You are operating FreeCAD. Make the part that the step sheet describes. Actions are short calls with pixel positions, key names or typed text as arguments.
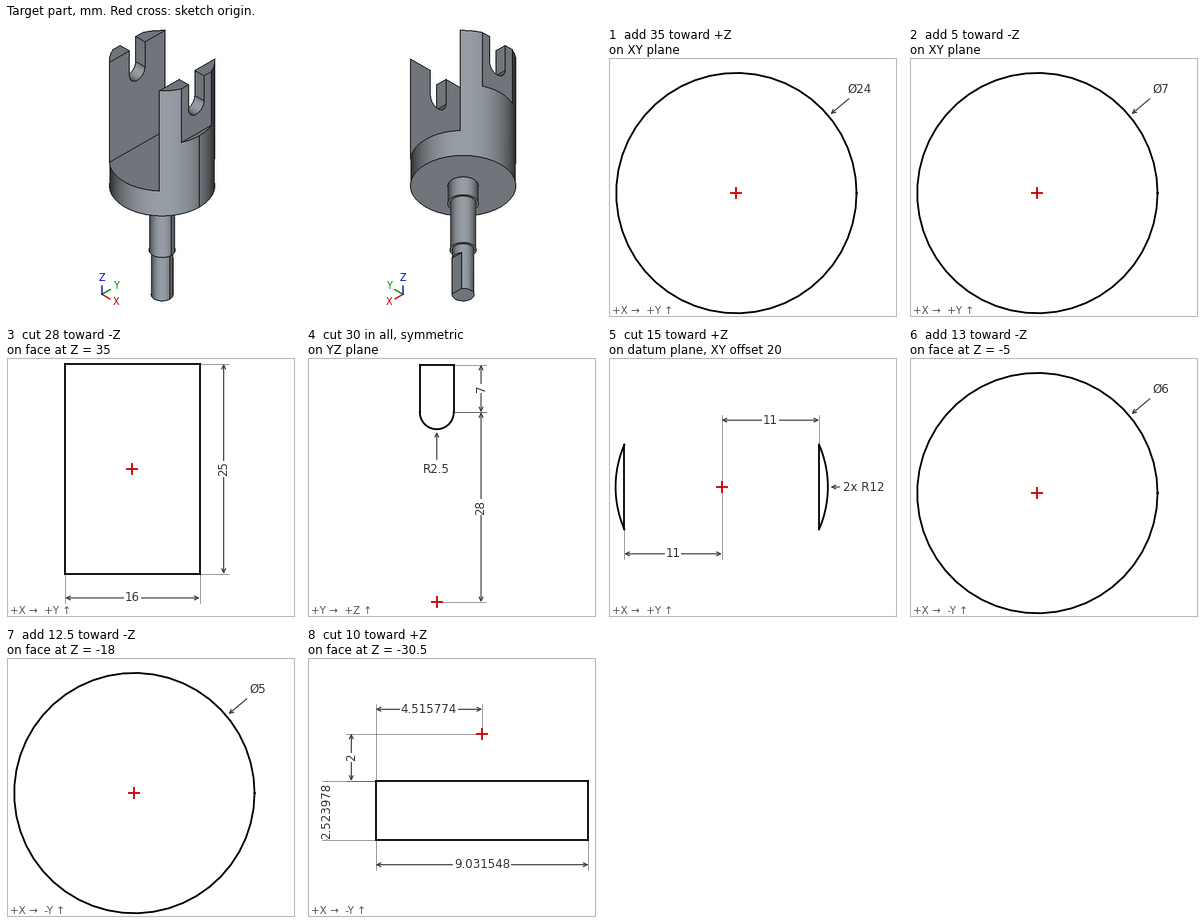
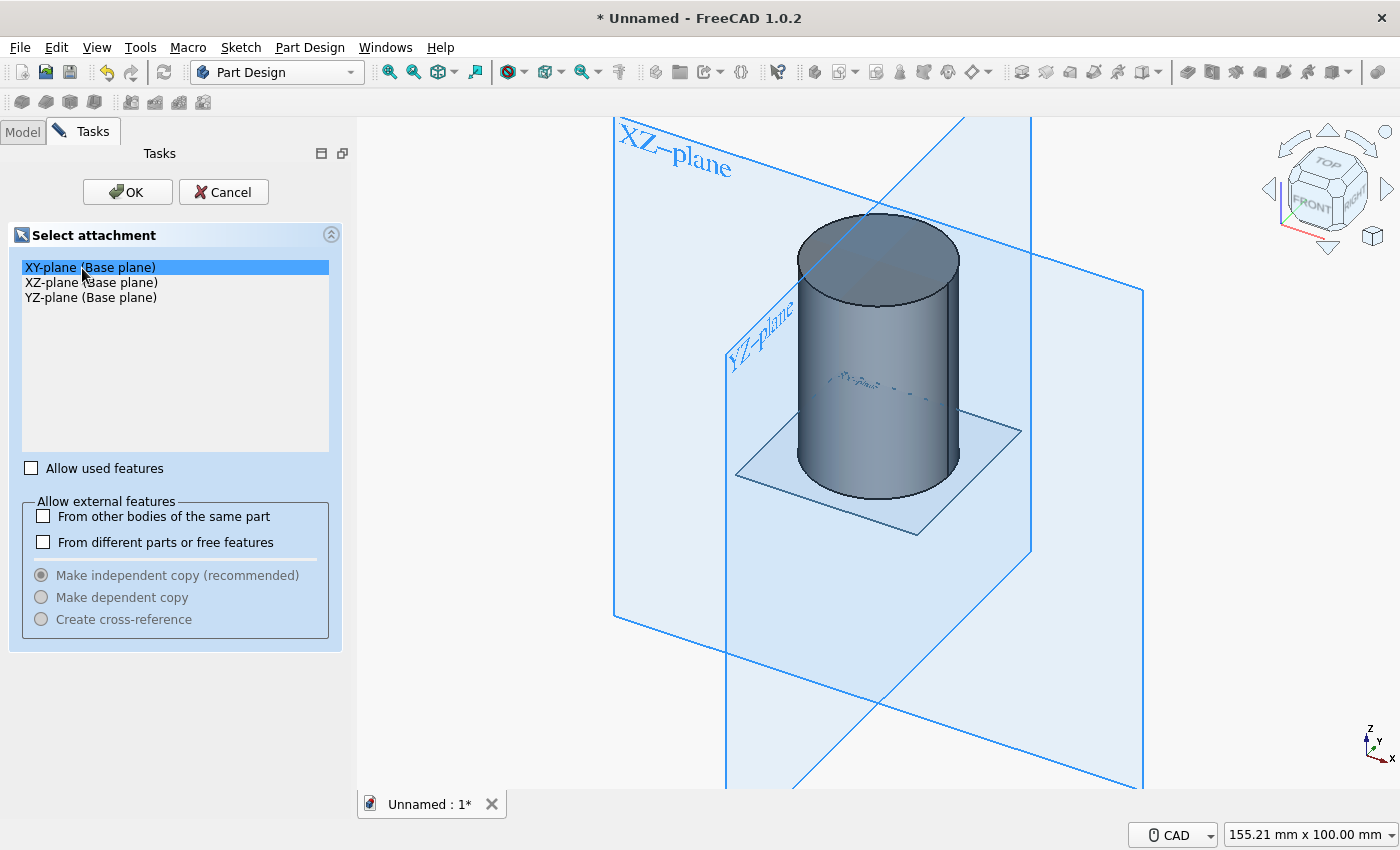
click(128, 192)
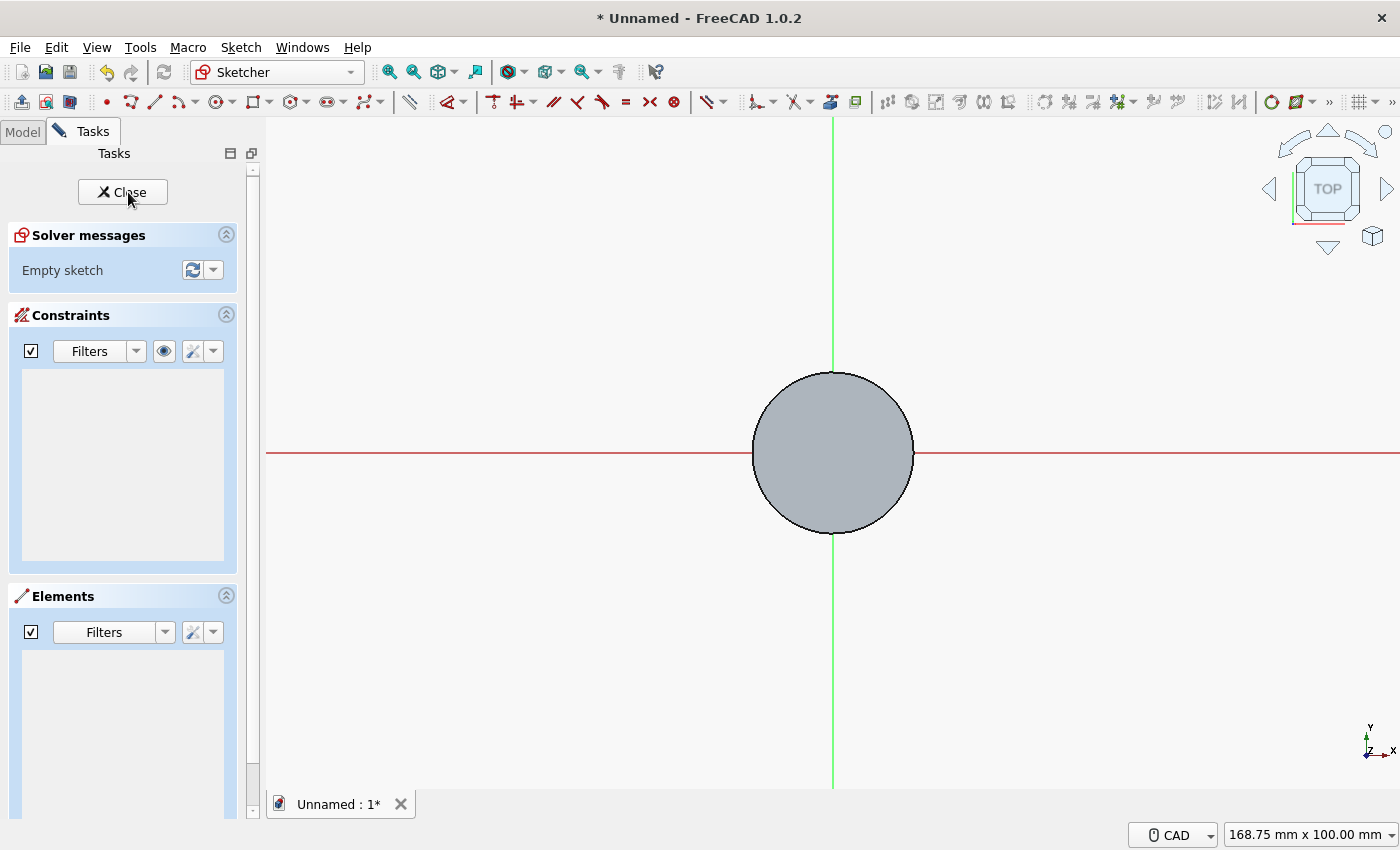
key(q)
key(s)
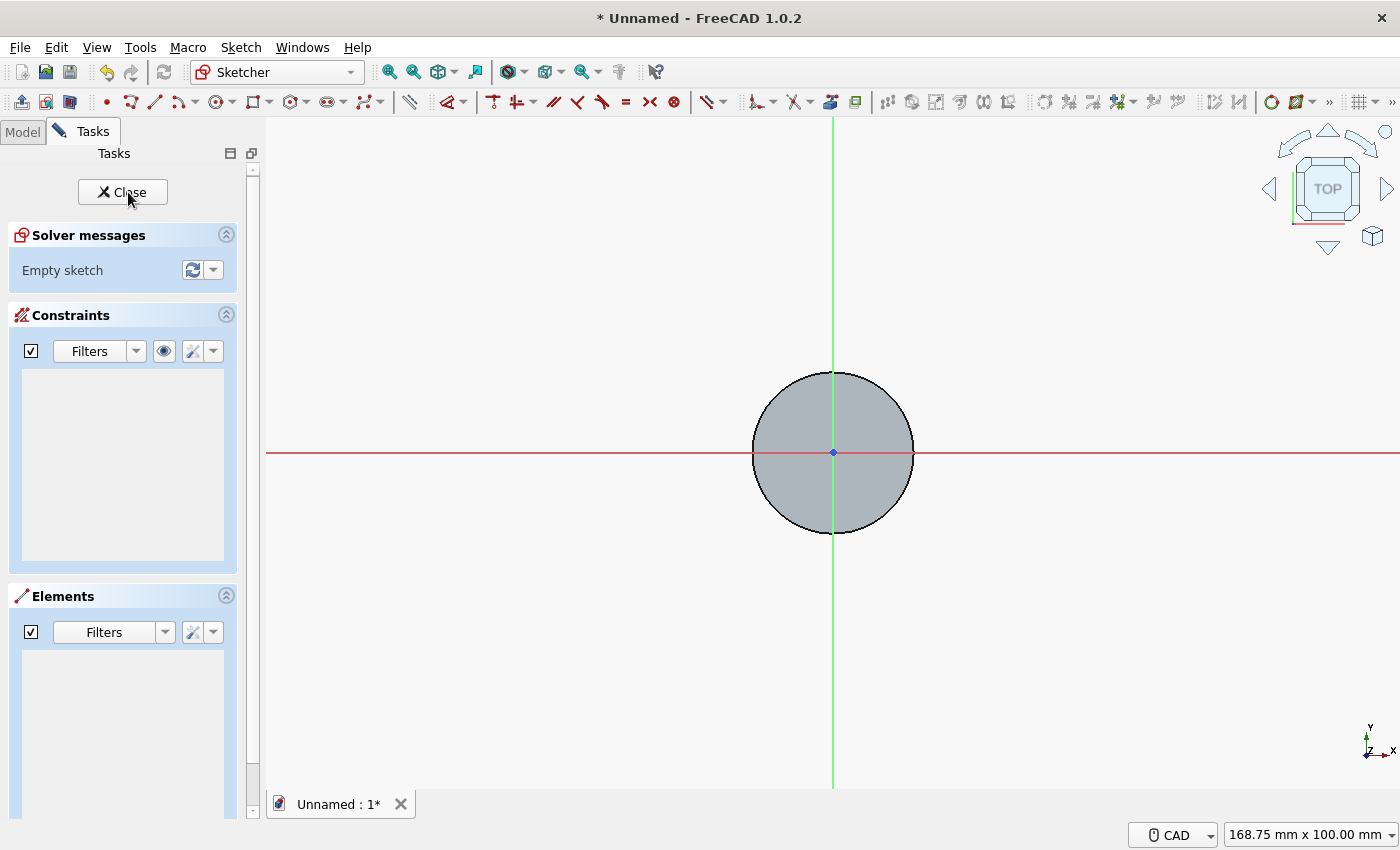
scroll(842, 453, up, 11)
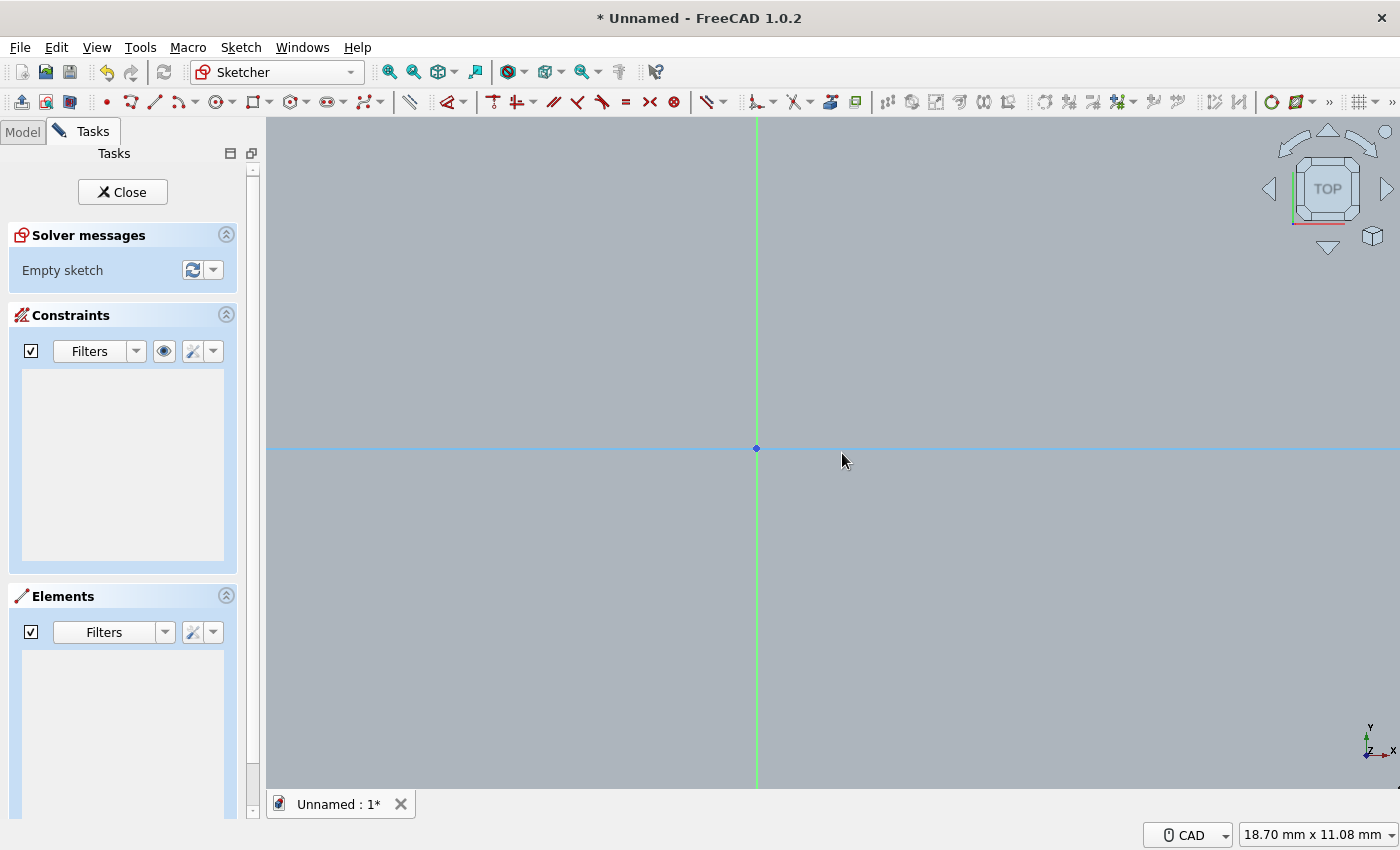
click(216, 102)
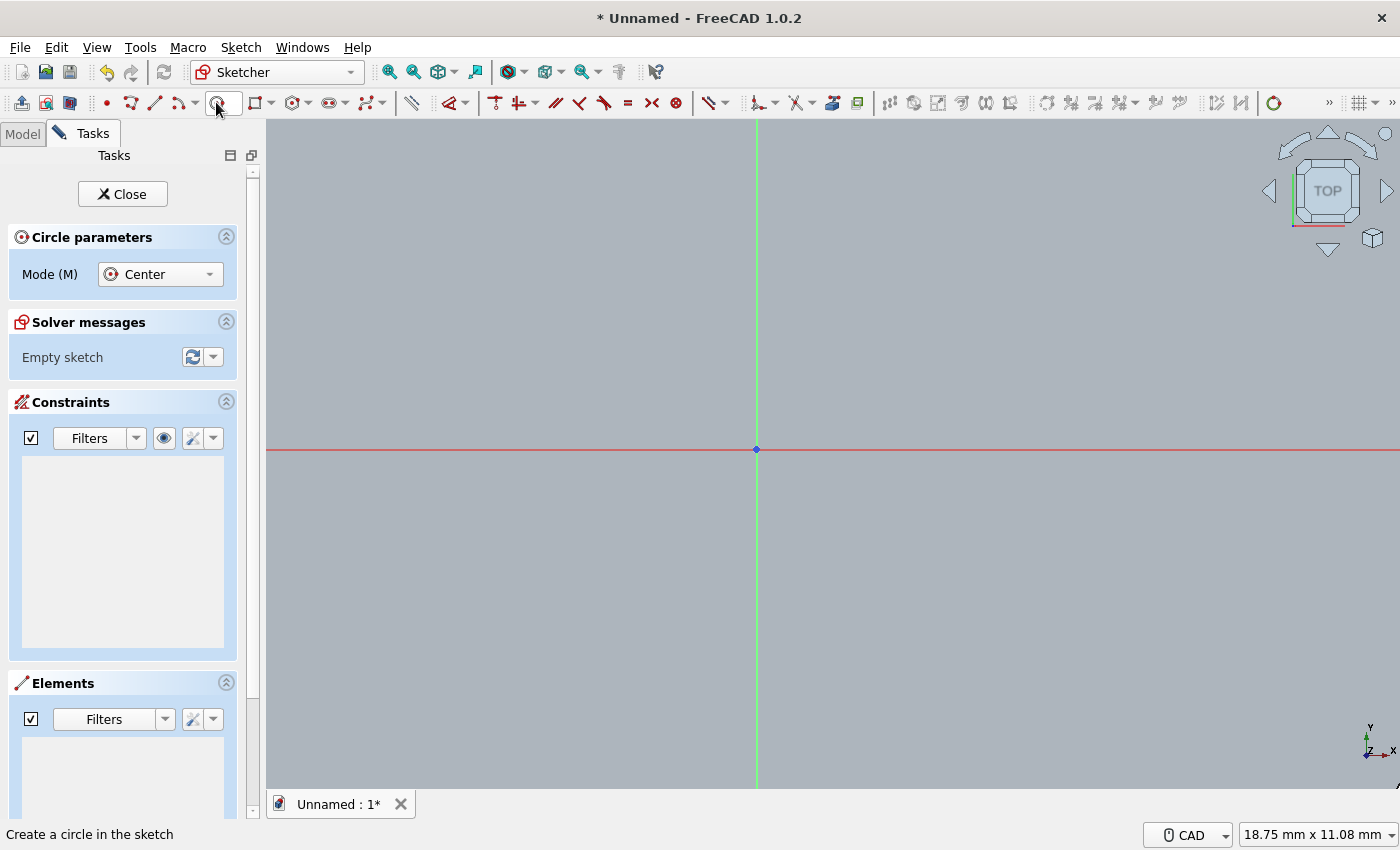
click(757, 450)
click(907, 300)
key(Escape)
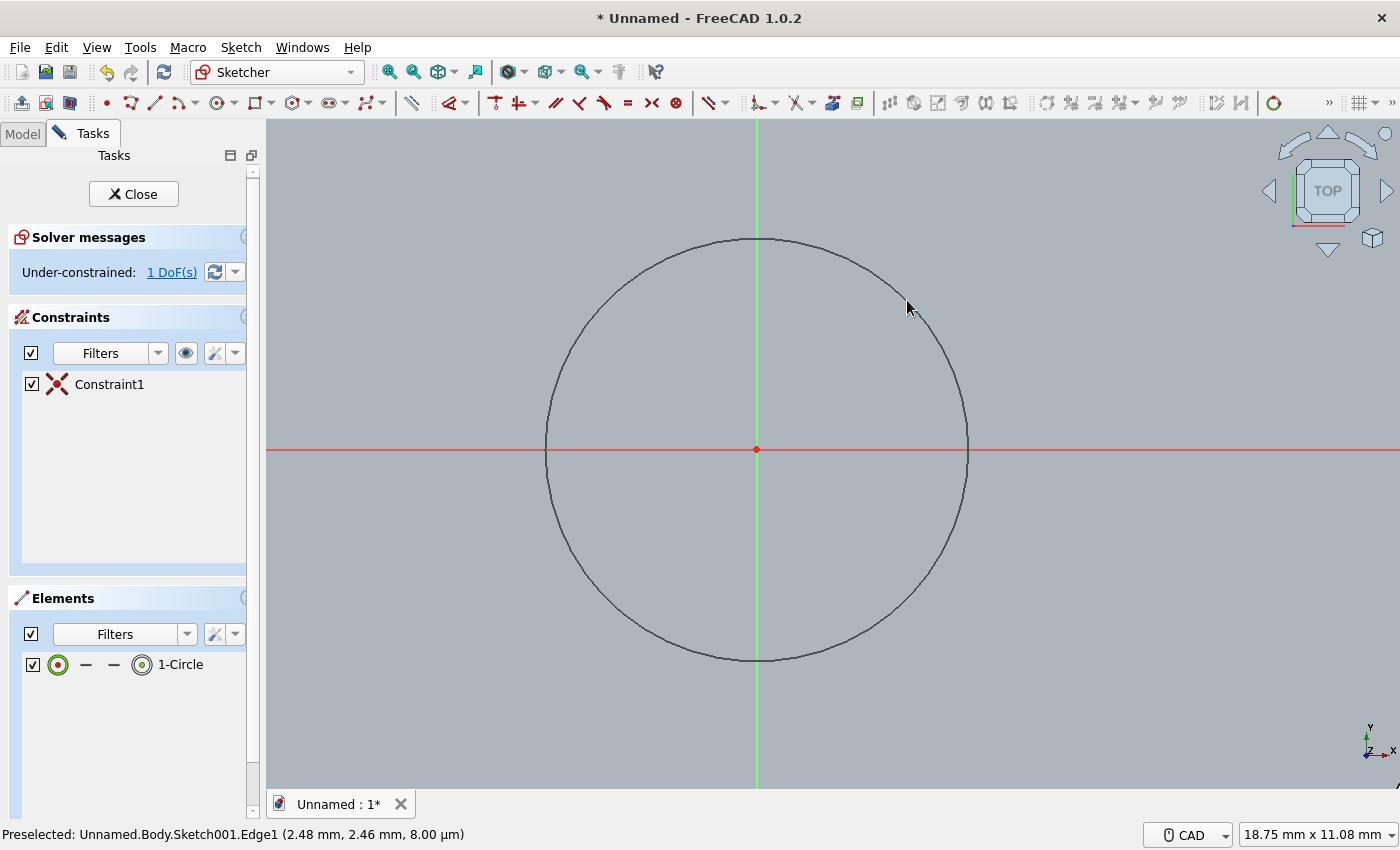
click(450, 104)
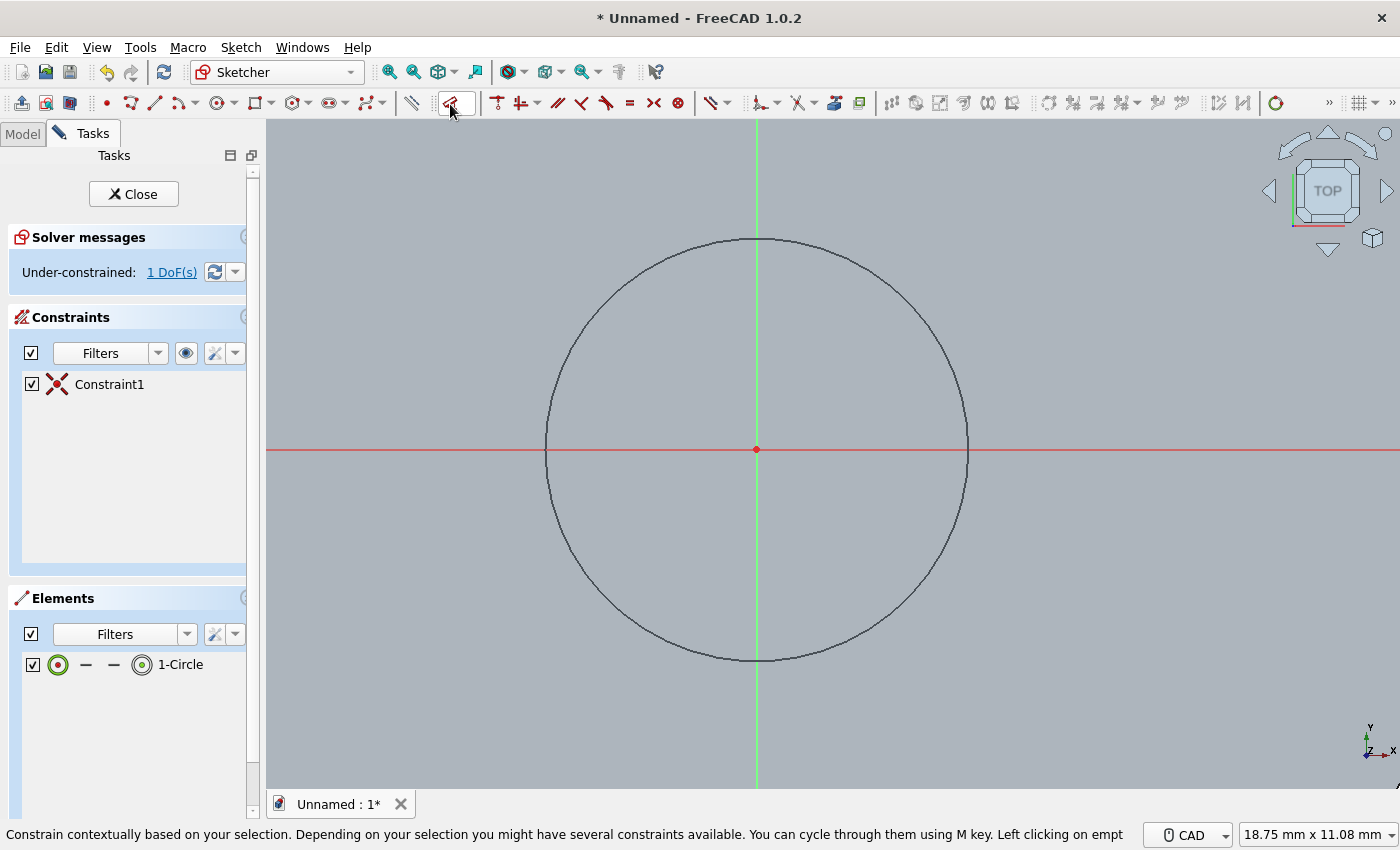
click(906, 300)
click(929, 277)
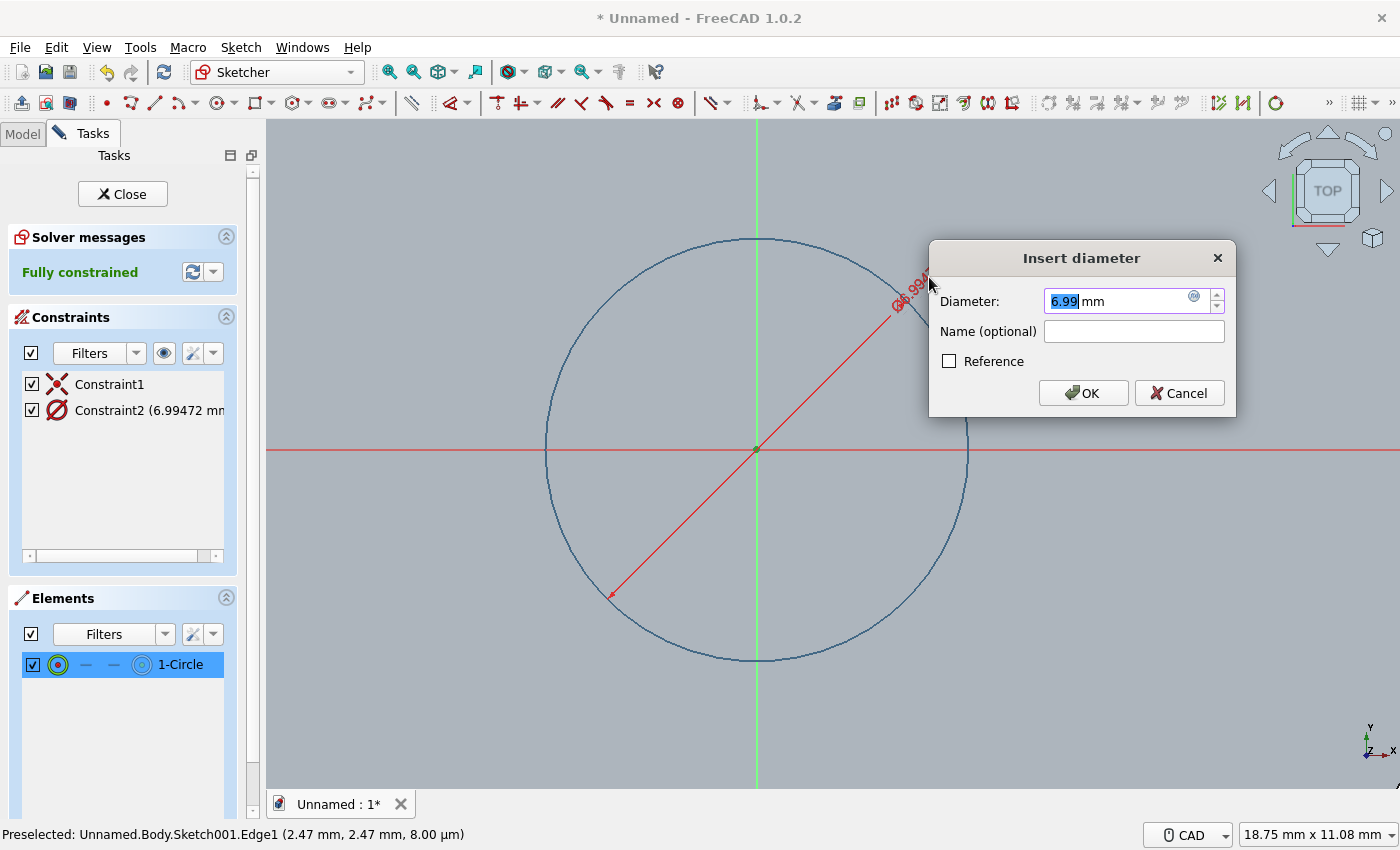
text(7)
key(Return)
key(Escape)